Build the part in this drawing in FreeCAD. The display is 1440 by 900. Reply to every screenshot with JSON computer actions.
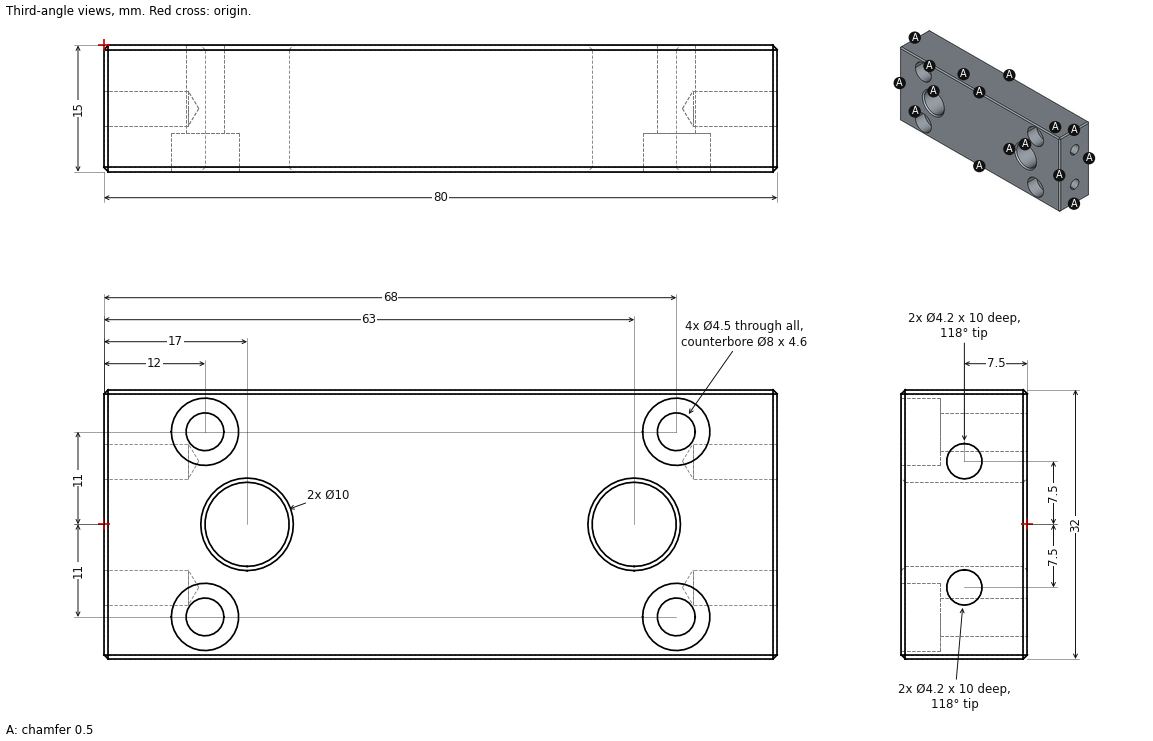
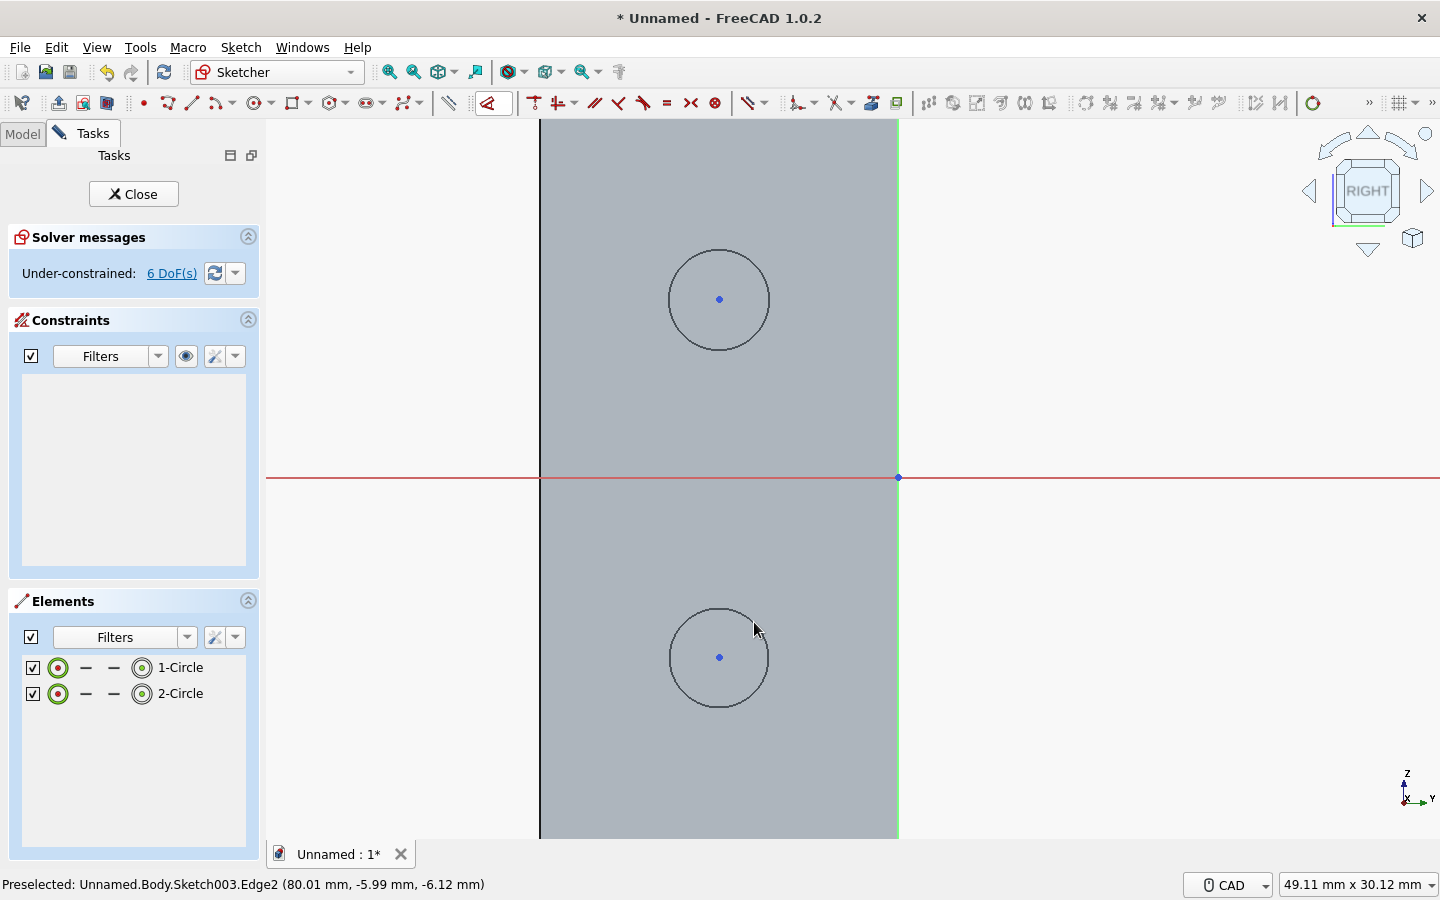
{"action": "left_click", "coordinate": [754, 264]}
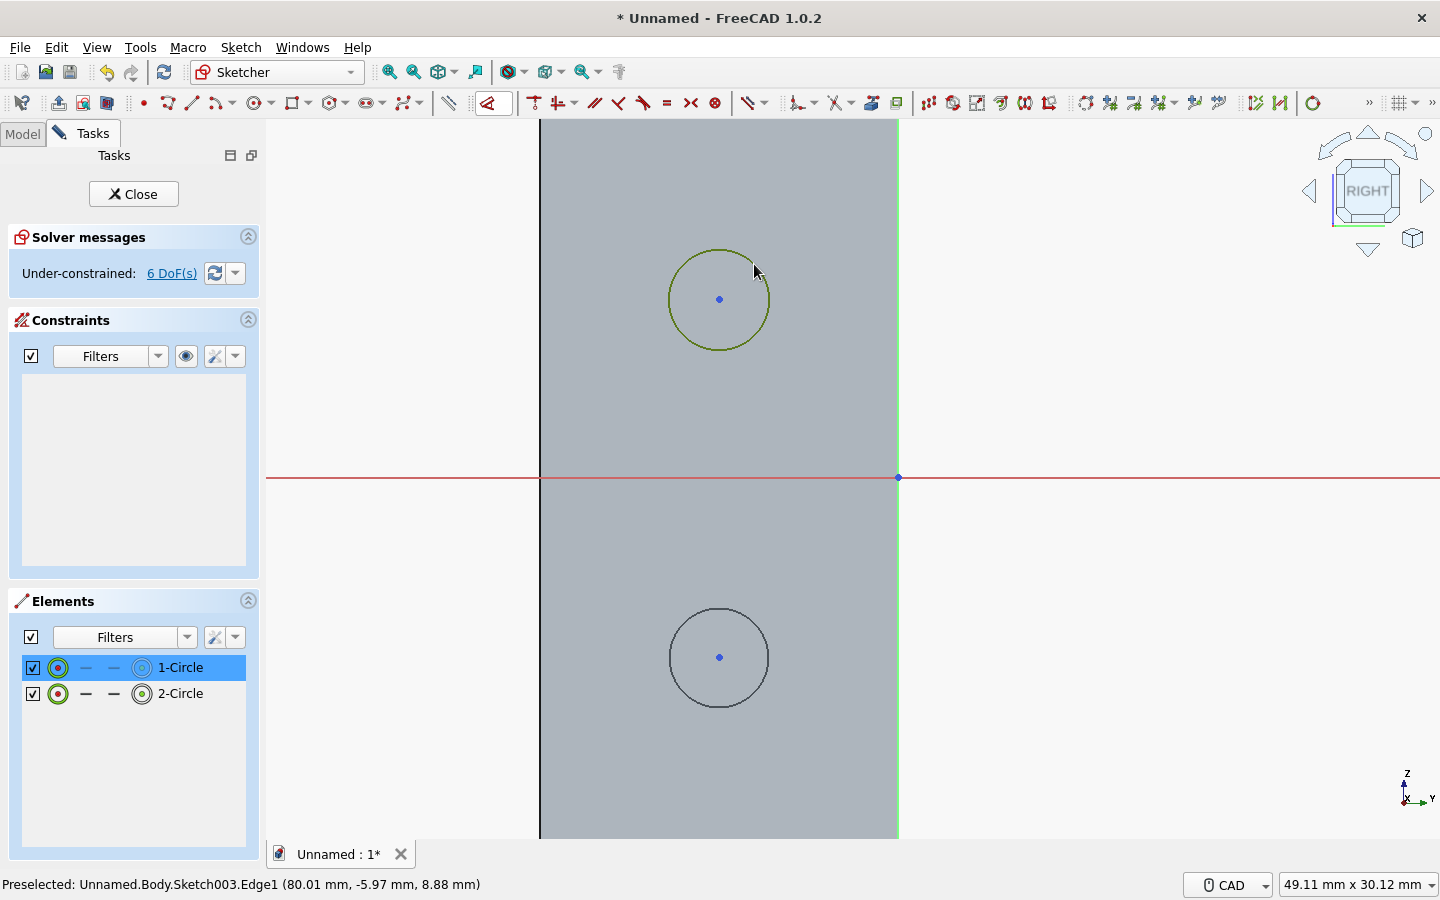
{"action": "left_click", "coordinate": [754, 623]}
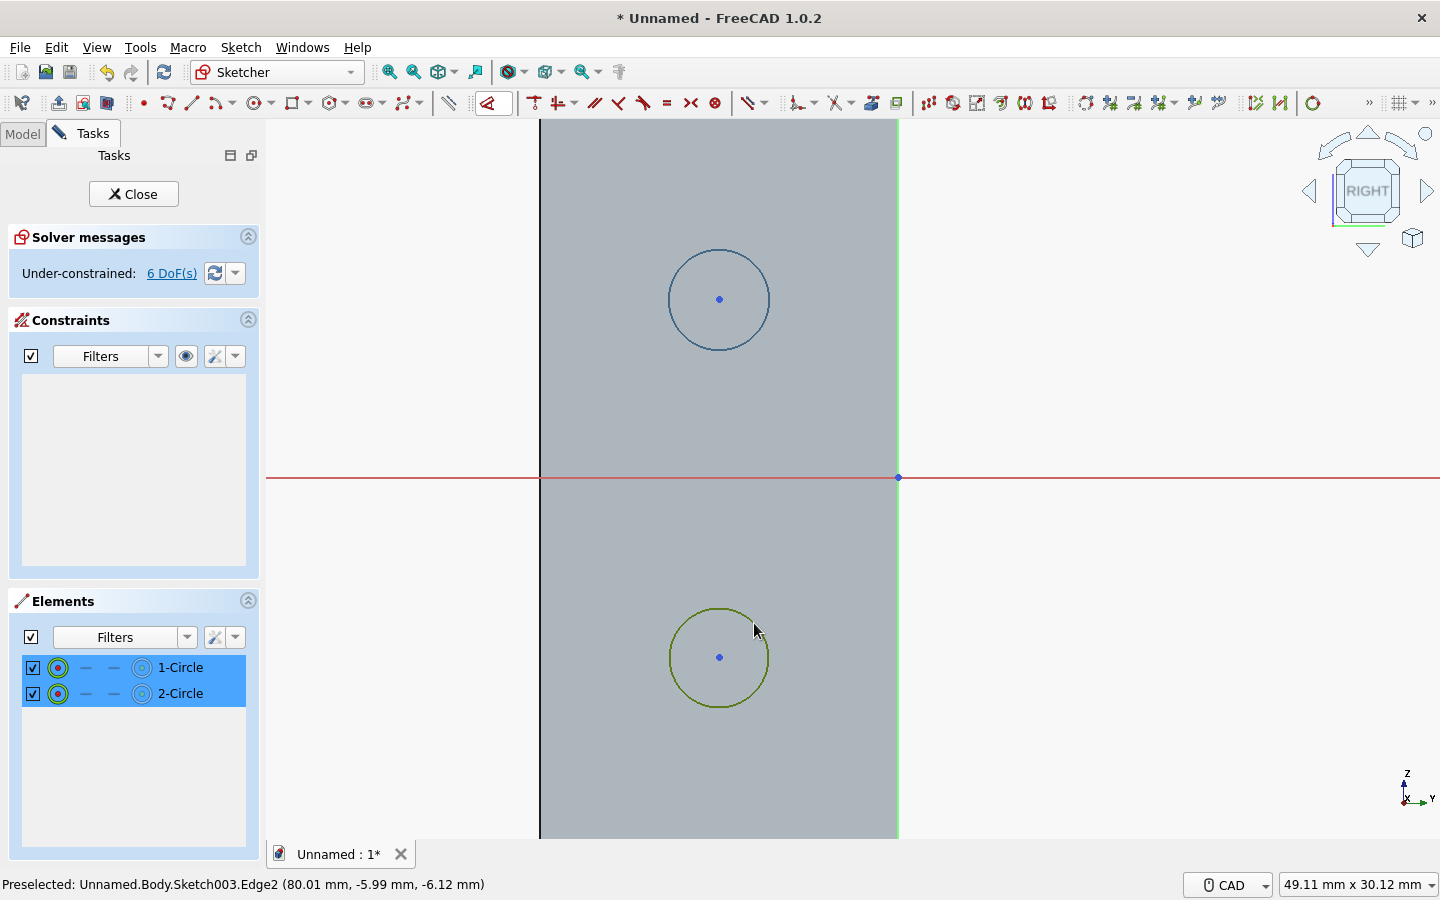
{"action": "left_click", "coordinate": [668, 104]}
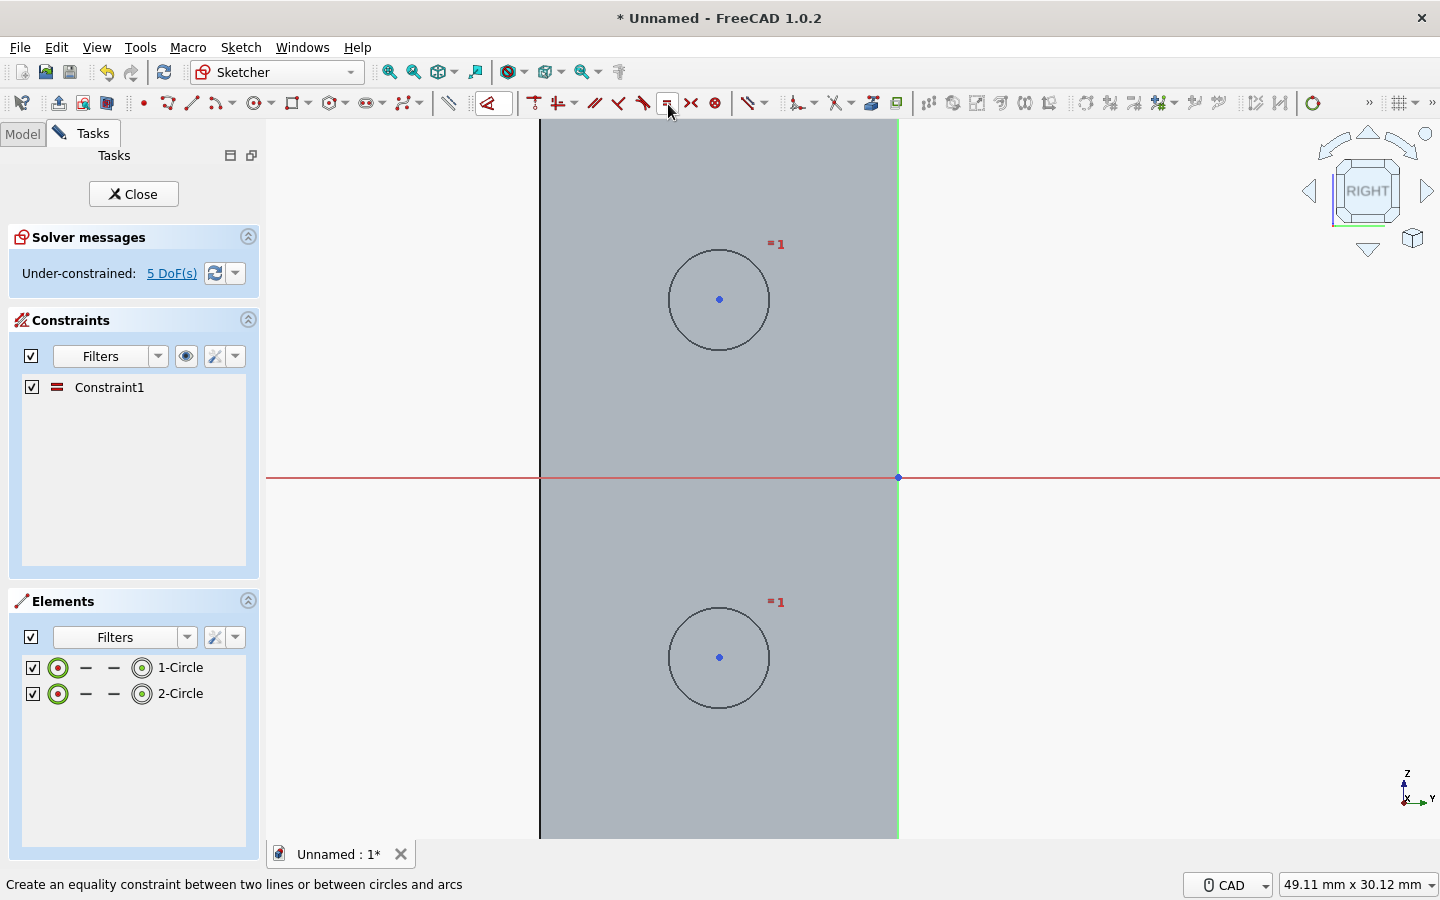
{"action": "left_click", "coordinate": [754, 264]}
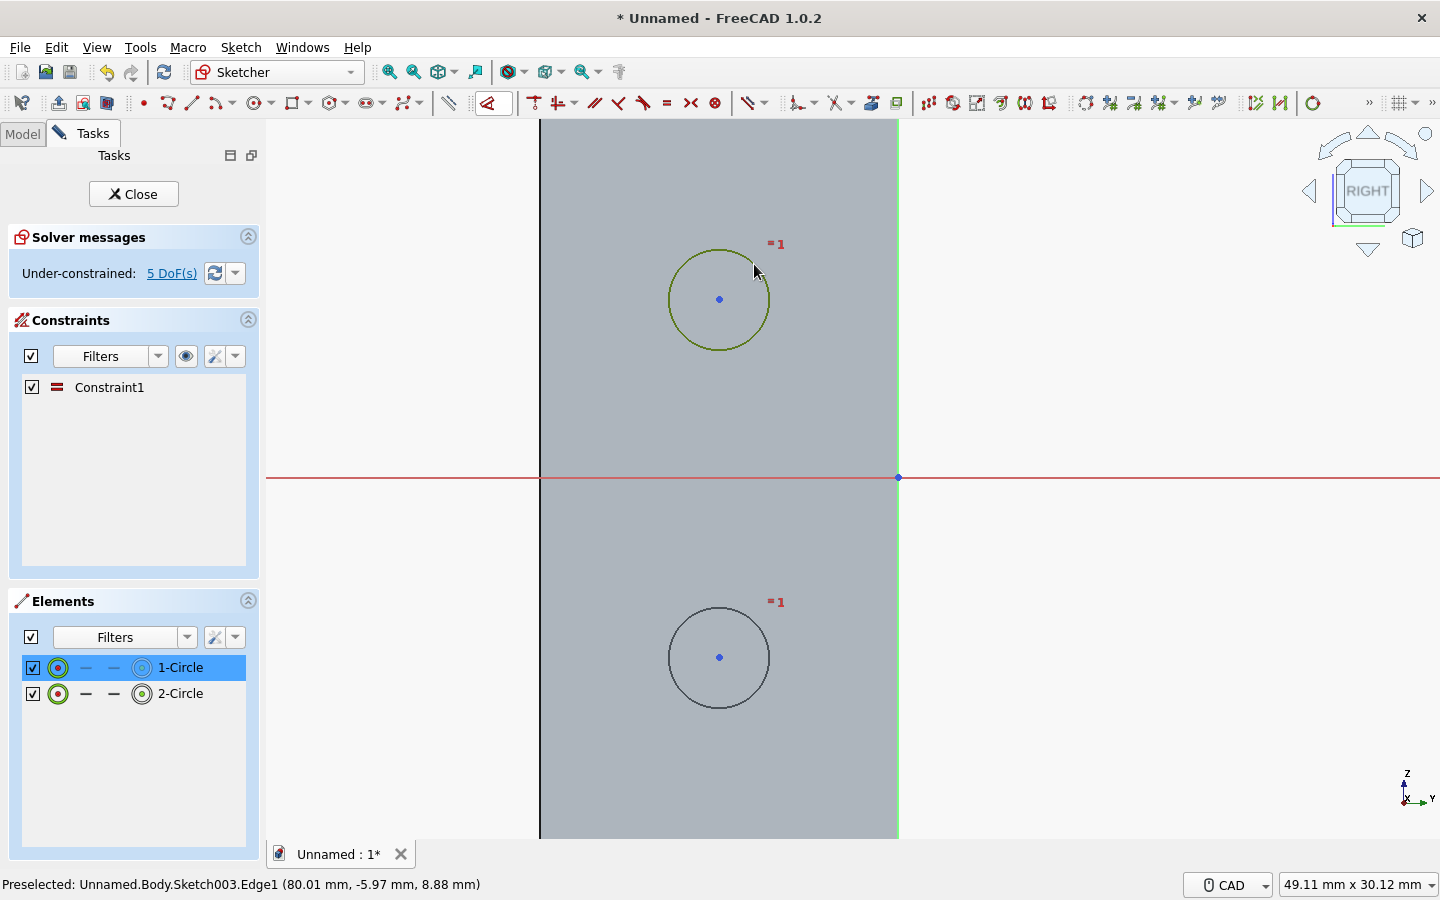
{"action": "key", "text": "k o"}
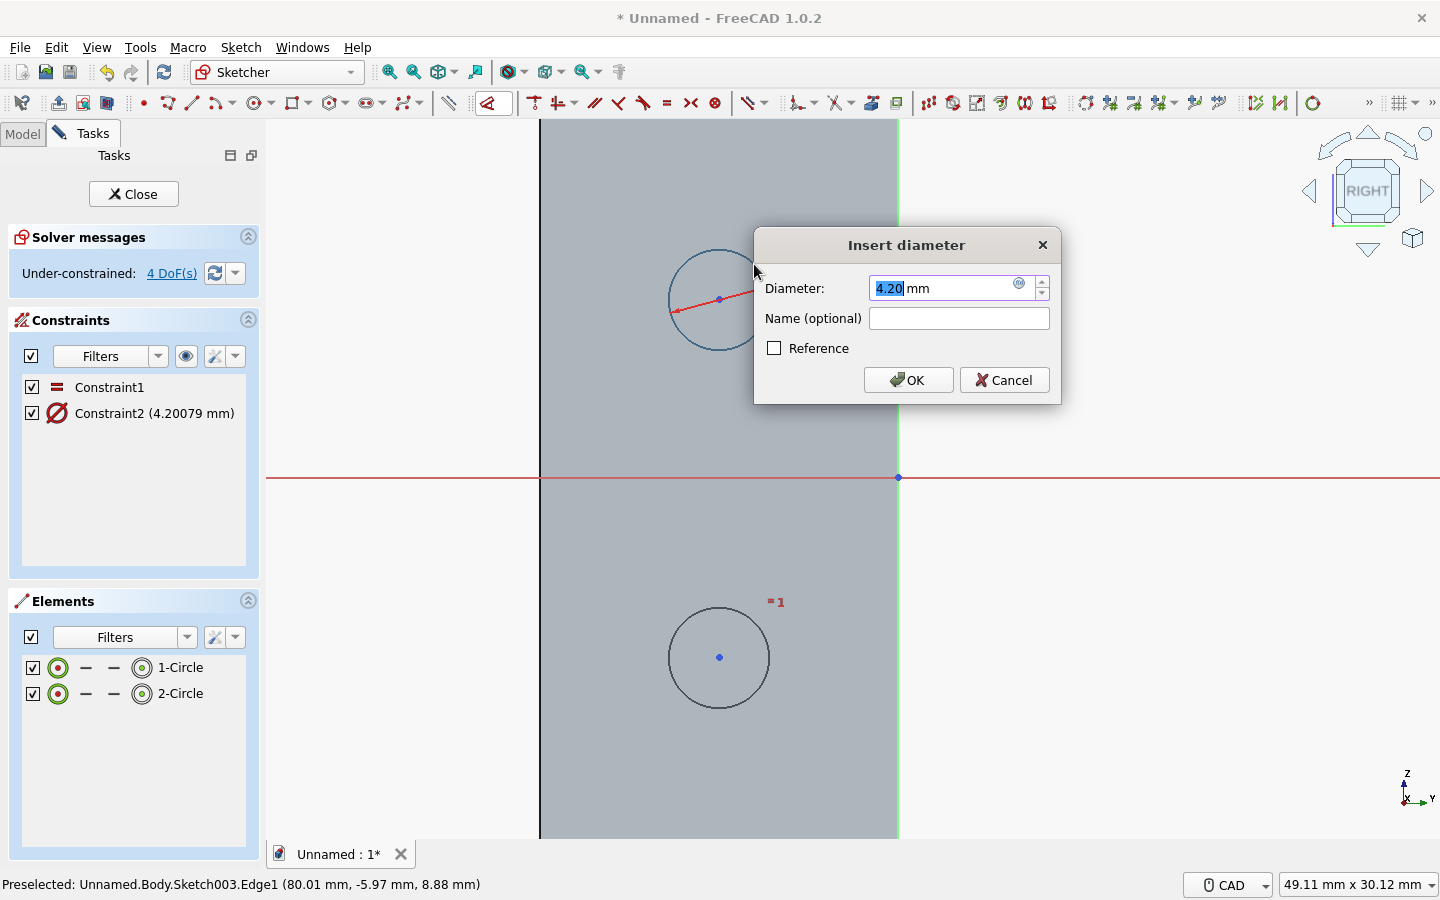
{"action": "type", "text": "4.2"}
{"action": "key", "text": "Return"}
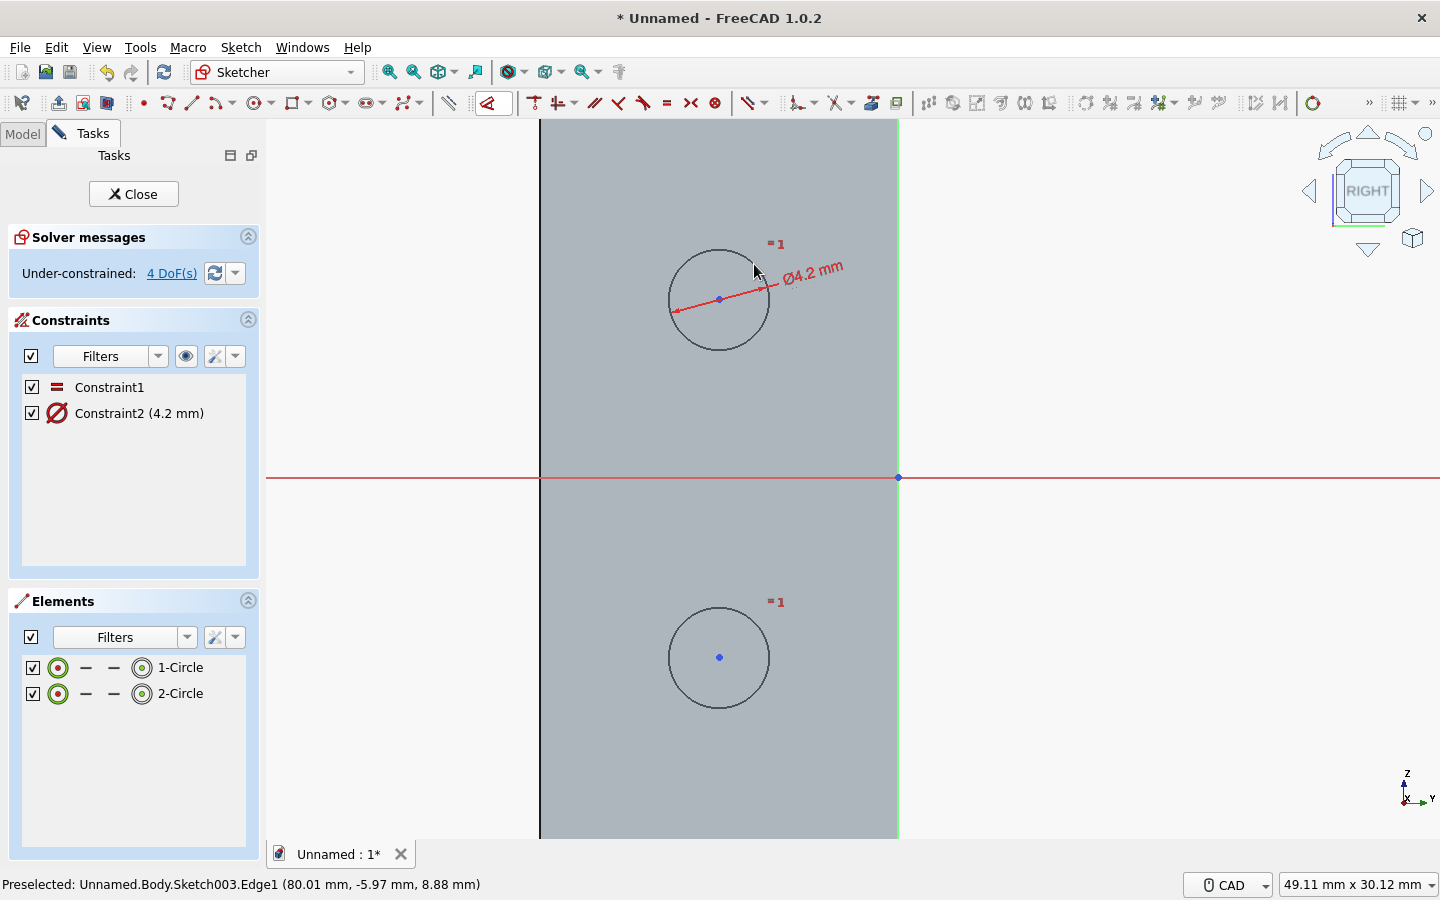
{"action": "left_click", "coordinate": [719, 300]}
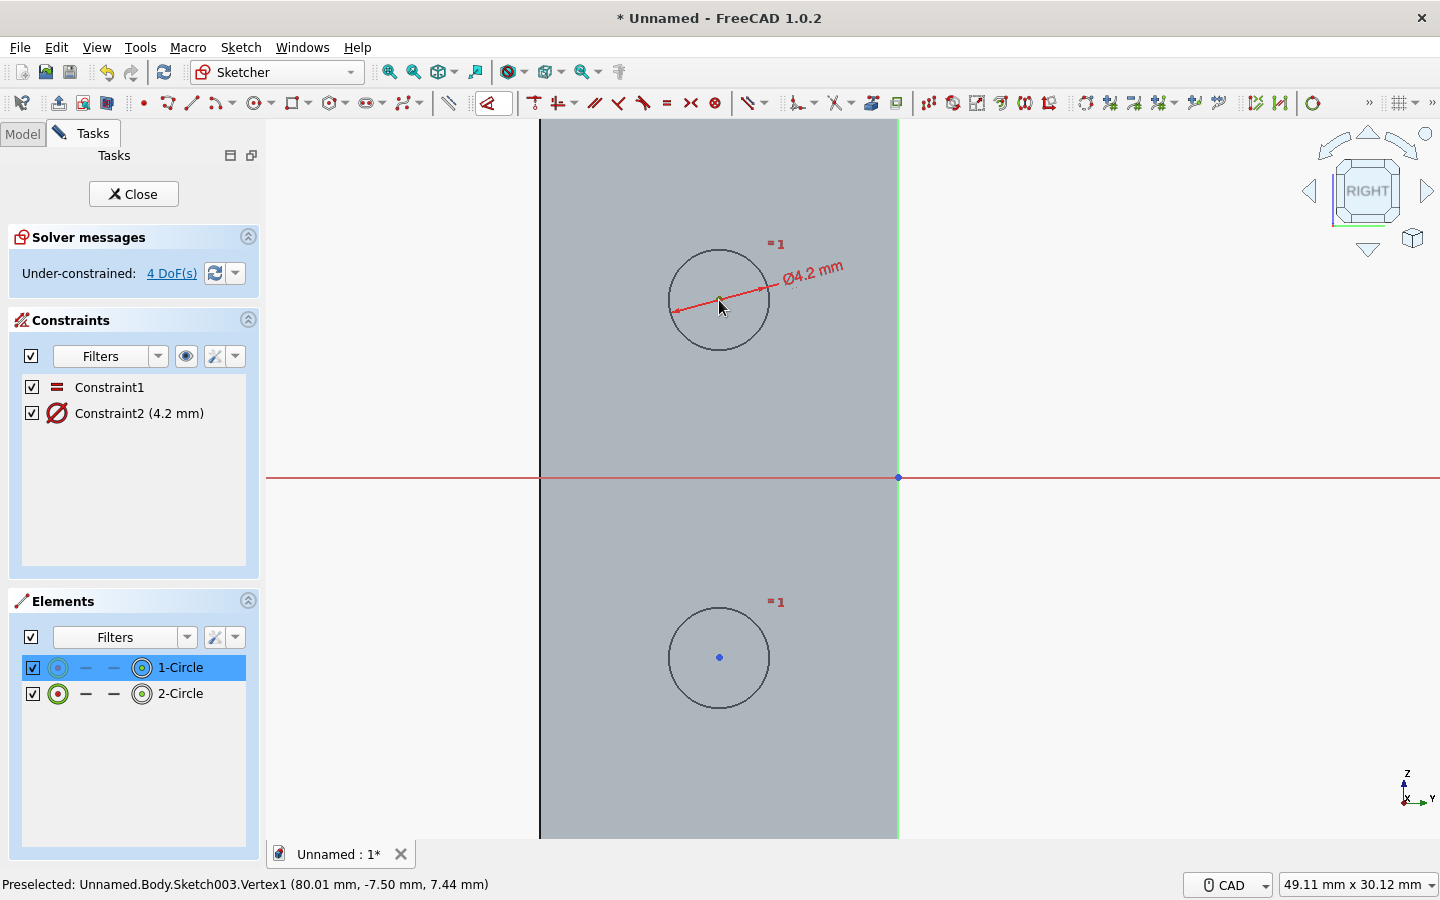
{"action": "left_click", "coordinate": [506, 104]}